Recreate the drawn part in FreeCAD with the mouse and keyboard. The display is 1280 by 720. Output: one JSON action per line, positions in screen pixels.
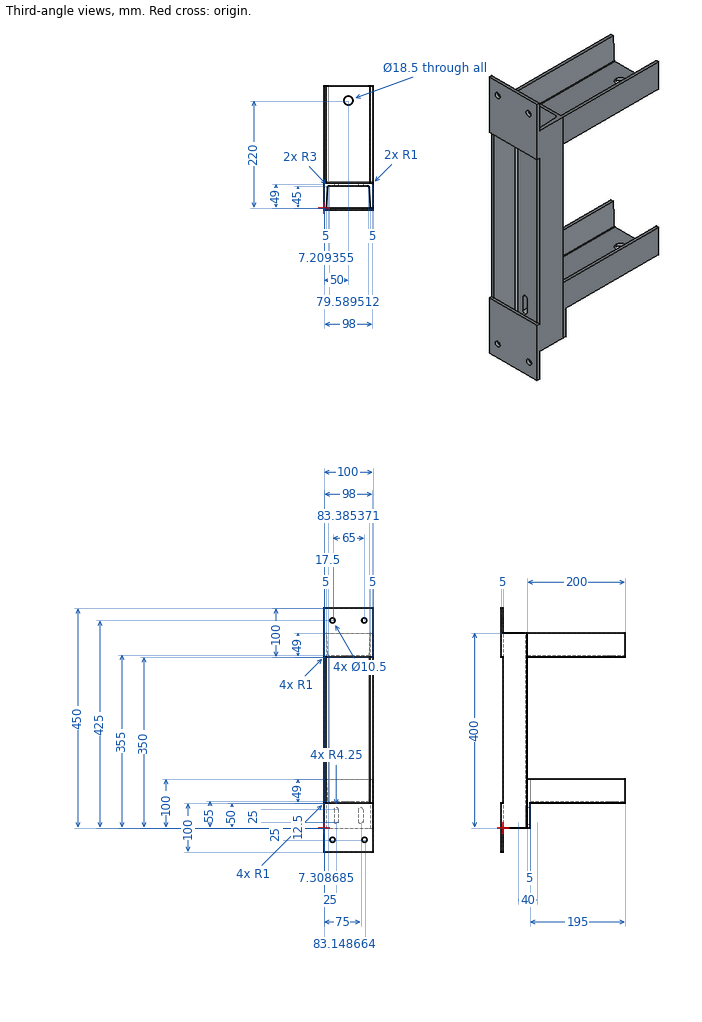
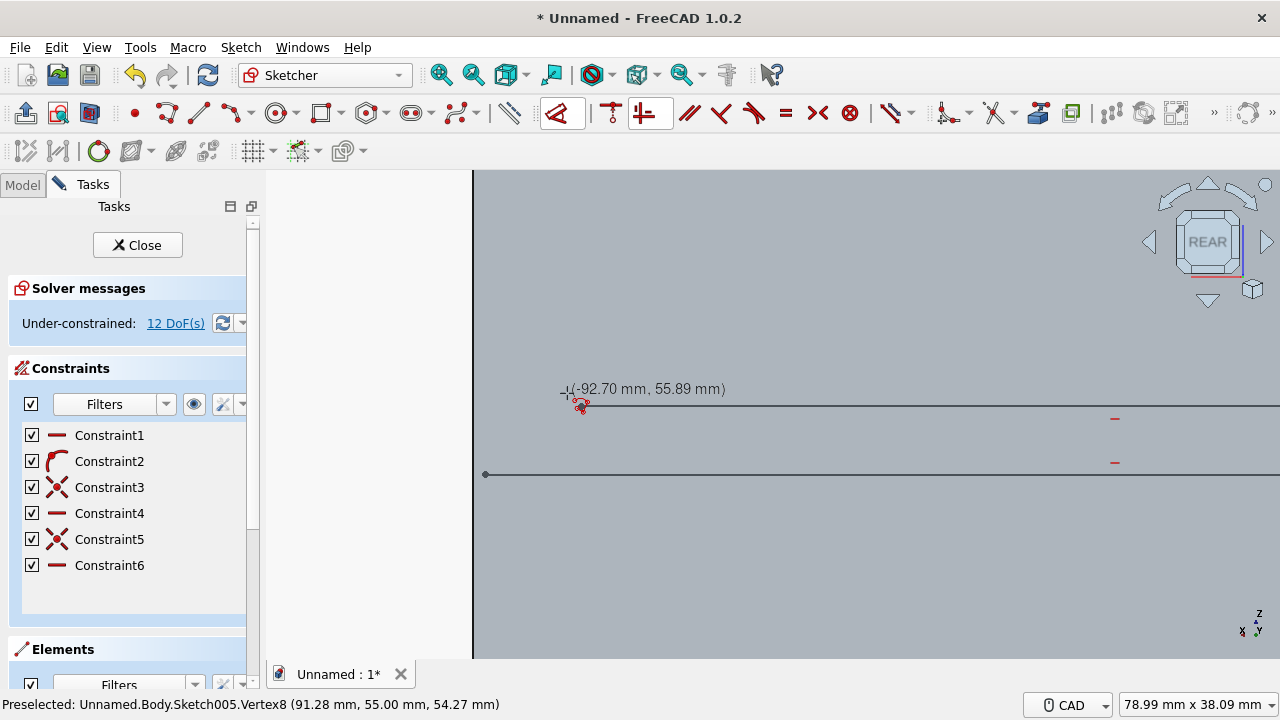
{"action": "scroll", "coordinate": [570, 396], "scroll_direction": "down", "scroll_amount": 7}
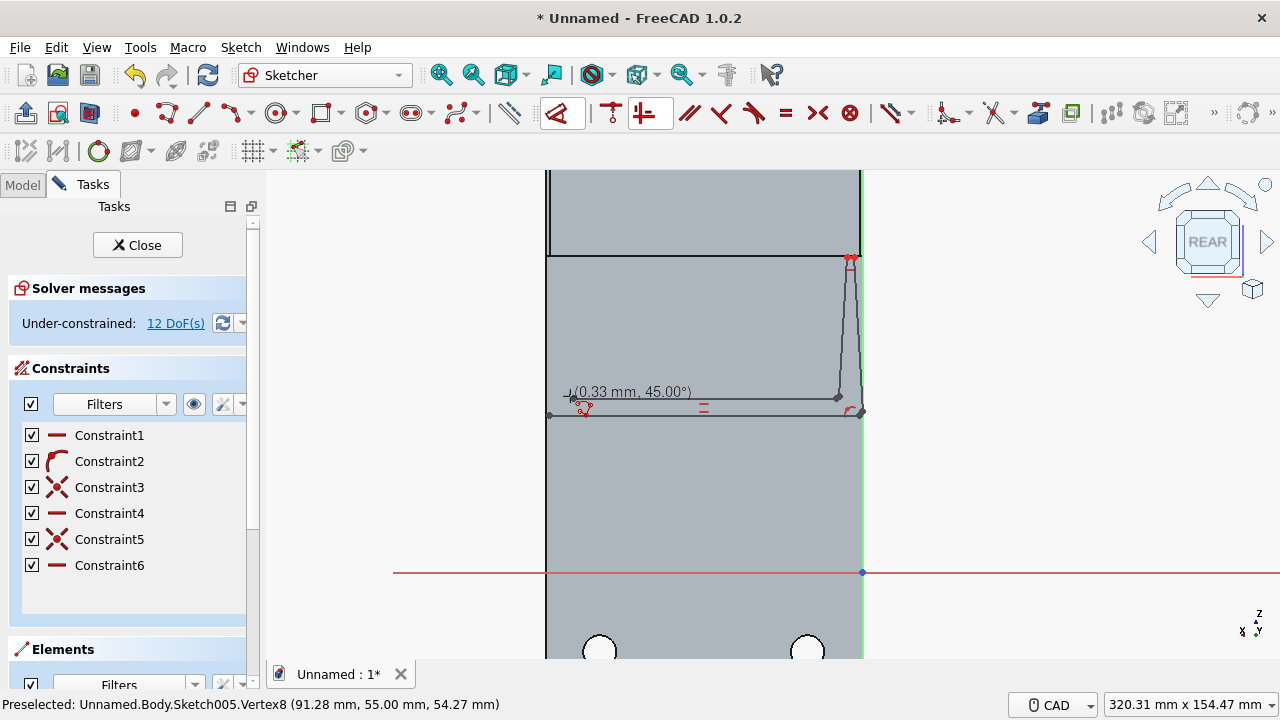
{"action": "left_click", "coordinate": [562, 256]}
{"action": "left_click", "coordinate": [546, 256]}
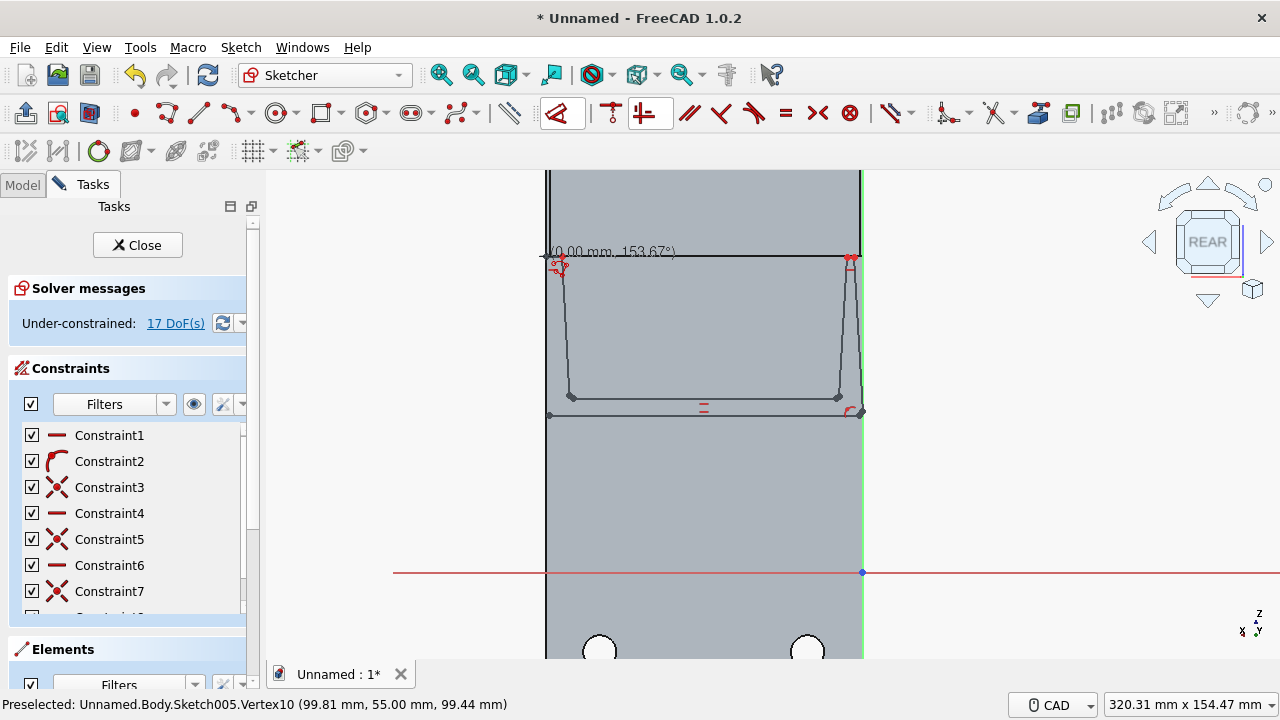
{"action": "scroll", "coordinate": [546, 411], "scroll_direction": "up", "scroll_amount": 7}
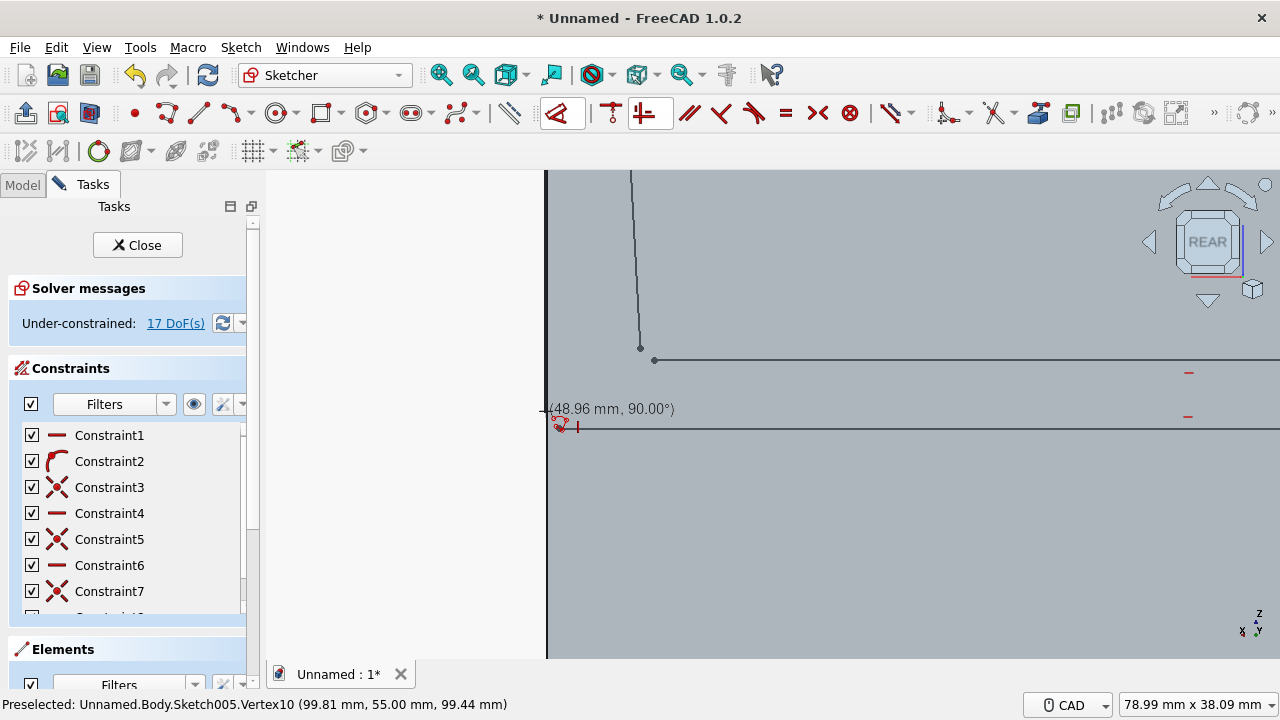
{"action": "left_click", "coordinate": [545, 411]}
{"action": "right_click", "coordinate": [545, 411]}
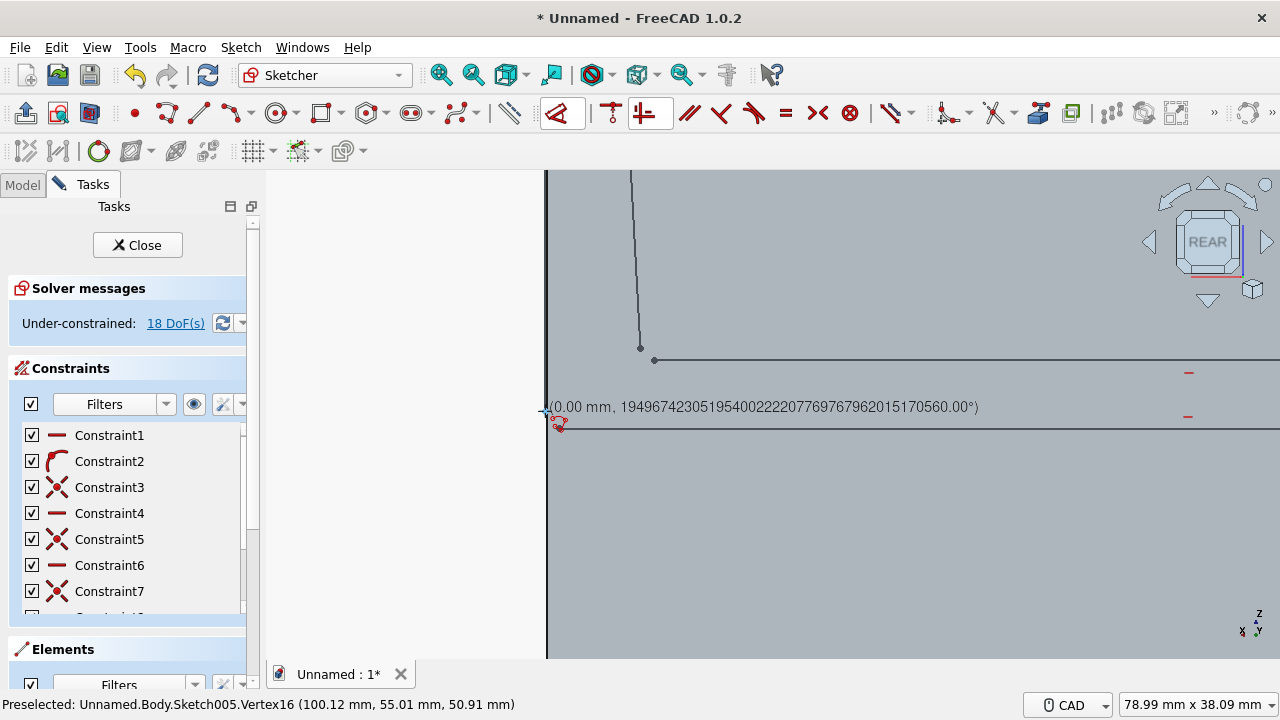
{"action": "key", "text": "g 3 a"}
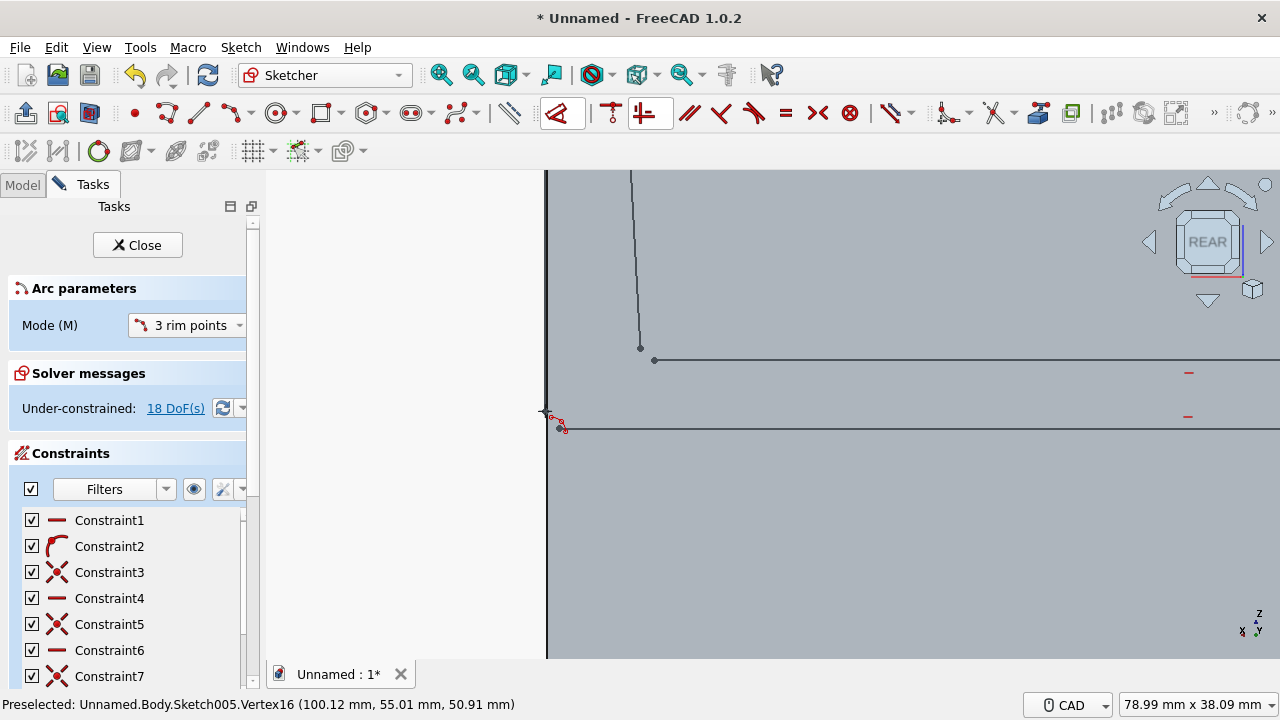
{"action": "scroll", "coordinate": [546, 411], "scroll_direction": "down", "scroll_amount": 7}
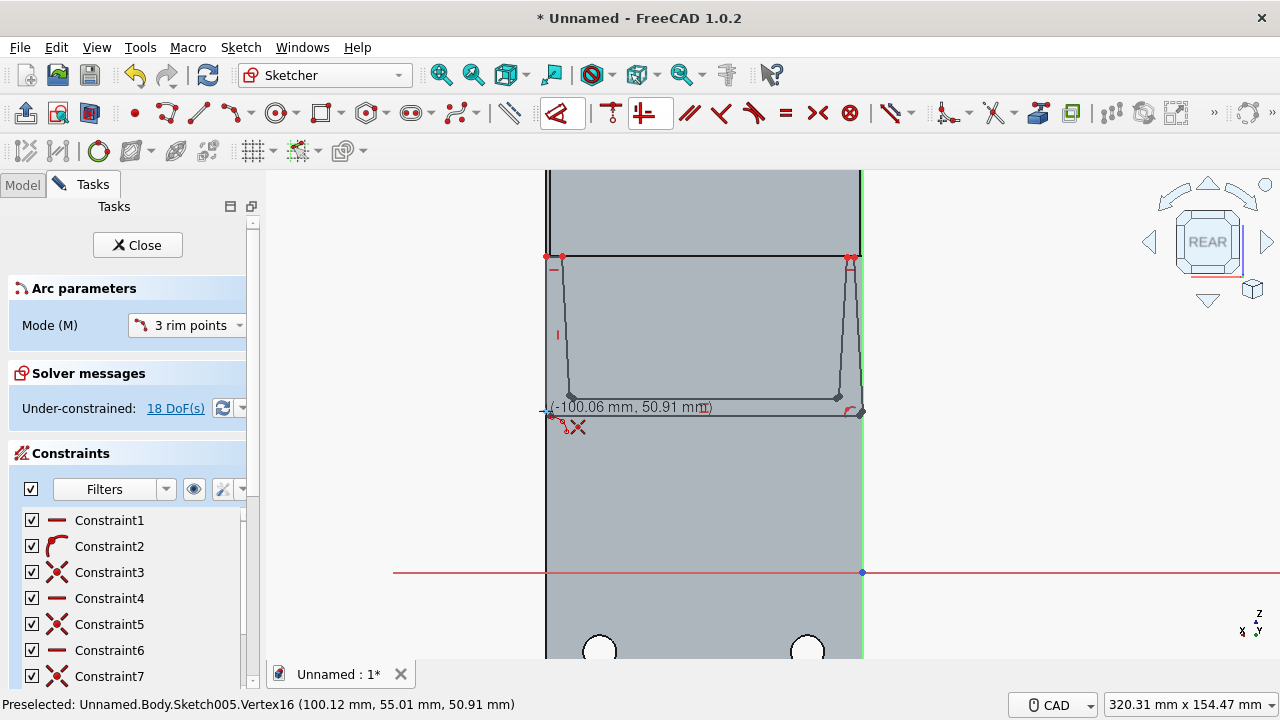
{"action": "scroll", "coordinate": [860, 415], "scroll_direction": "up", "scroll_amount": 9}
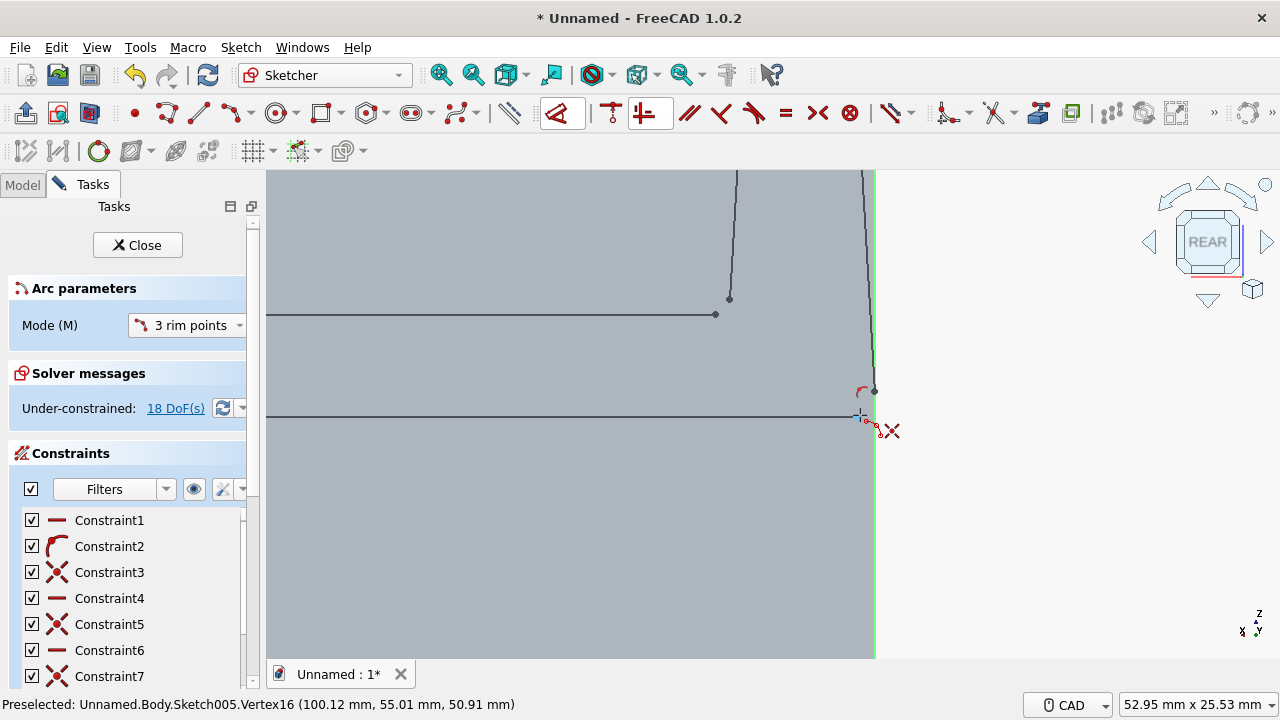
{"action": "left_click", "coordinate": [856, 417]}
{"action": "left_click", "coordinate": [875, 391]}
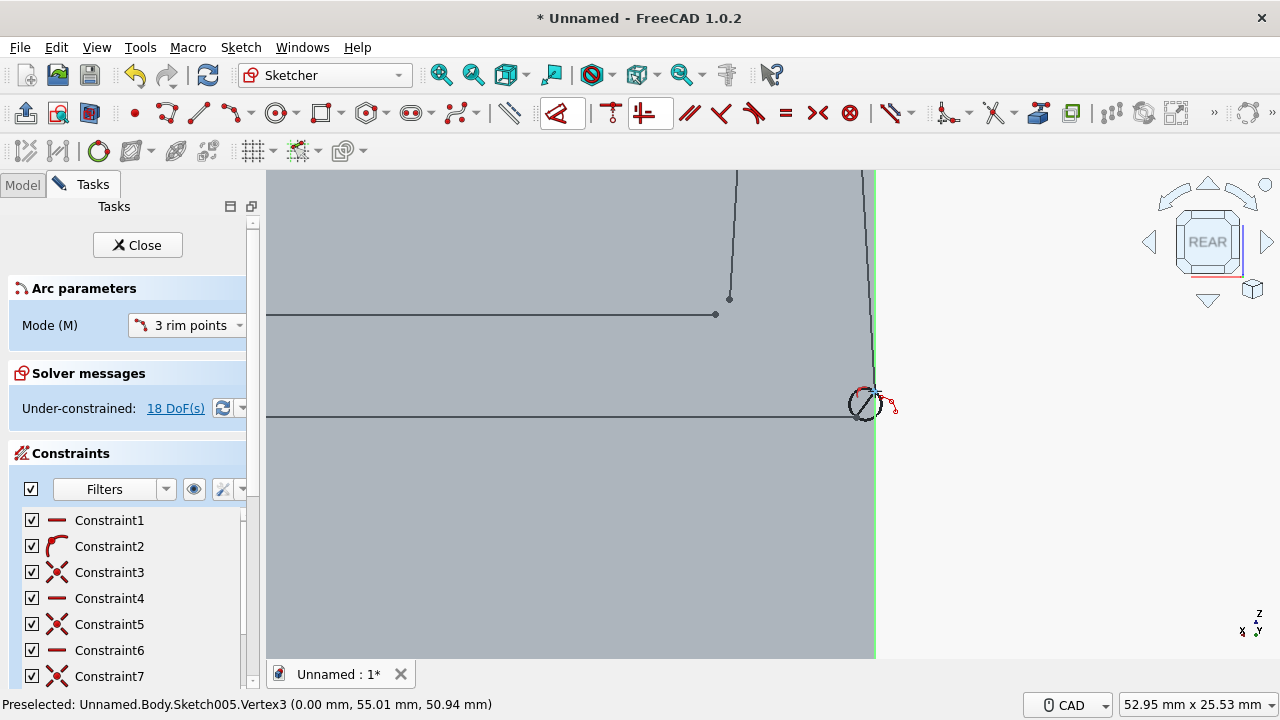
{"action": "scroll", "coordinate": [869, 404], "scroll_direction": "up", "scroll_amount": 6}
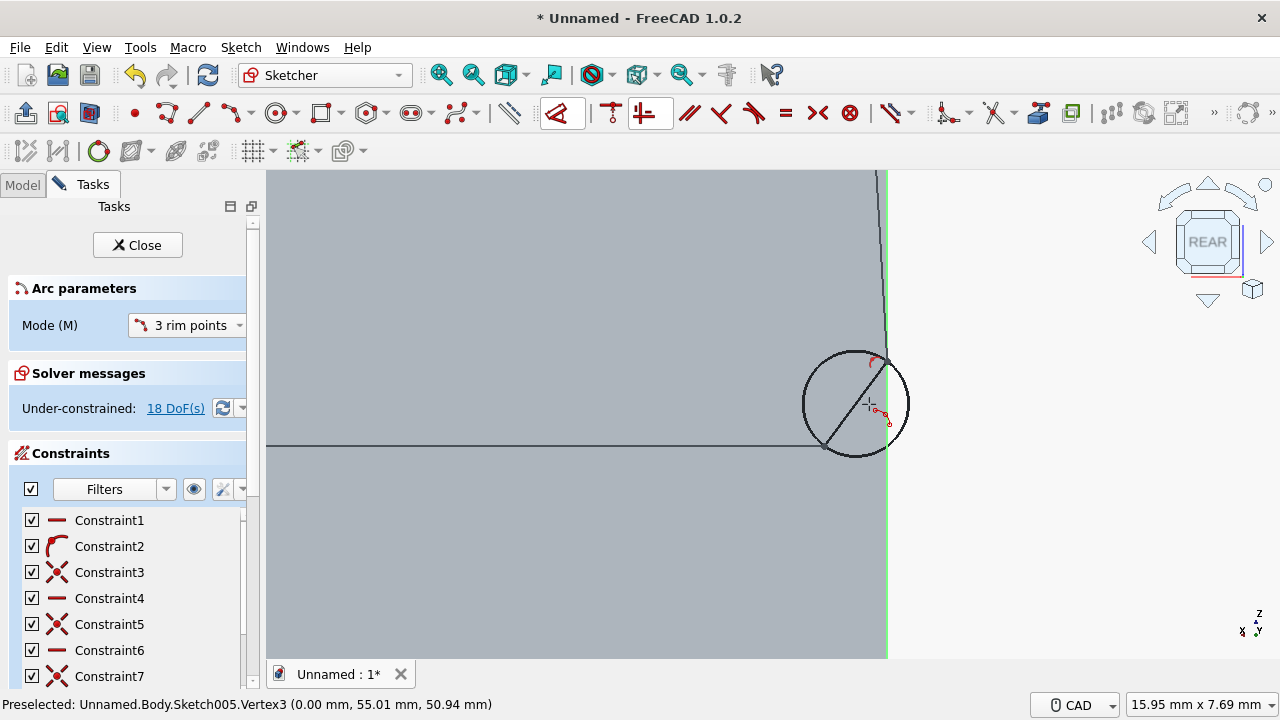
{"action": "left_click", "coordinate": [869, 402]}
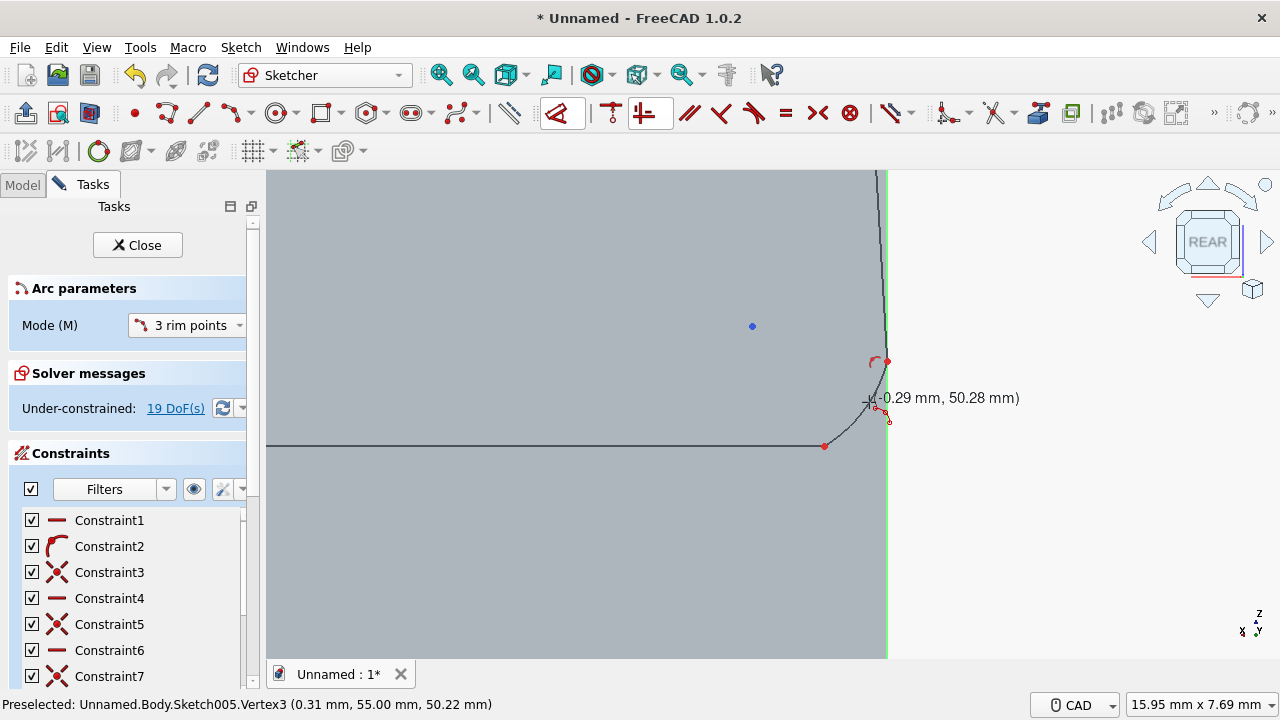
{"action": "scroll", "coordinate": [861, 414], "scroll_direction": "down", "scroll_amount": 15}